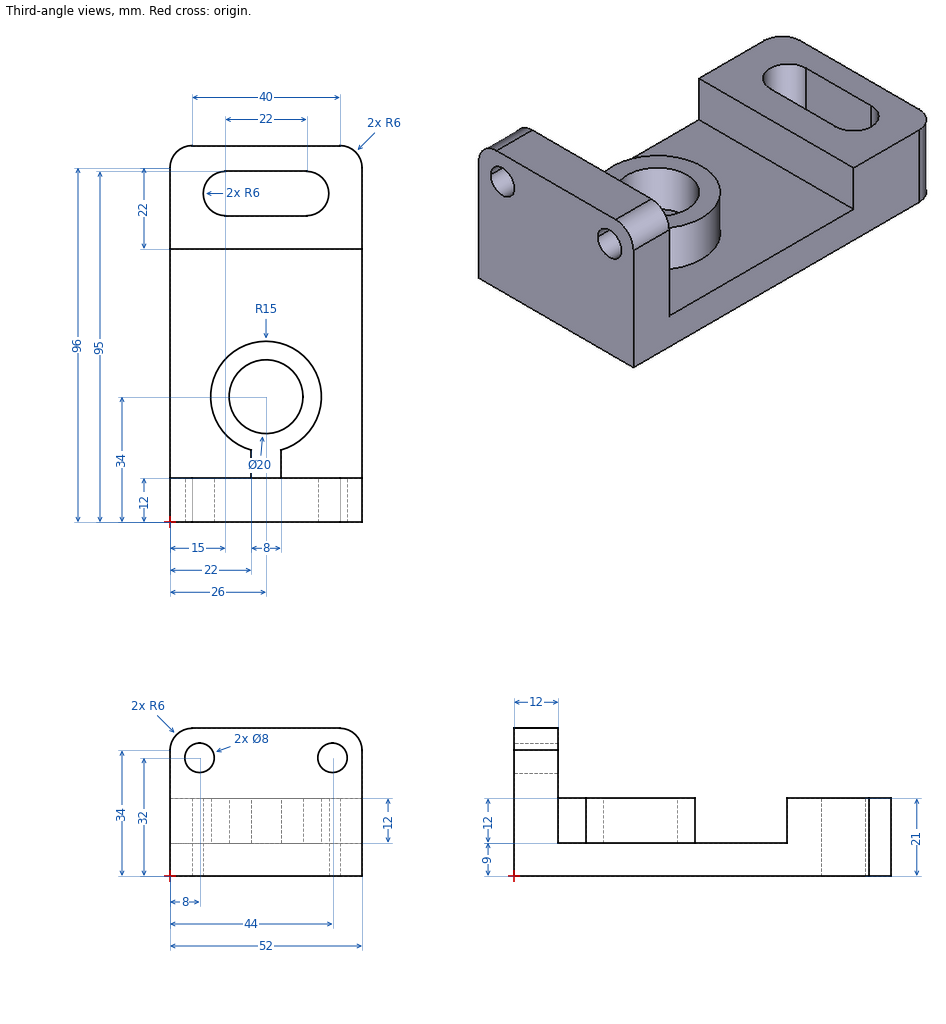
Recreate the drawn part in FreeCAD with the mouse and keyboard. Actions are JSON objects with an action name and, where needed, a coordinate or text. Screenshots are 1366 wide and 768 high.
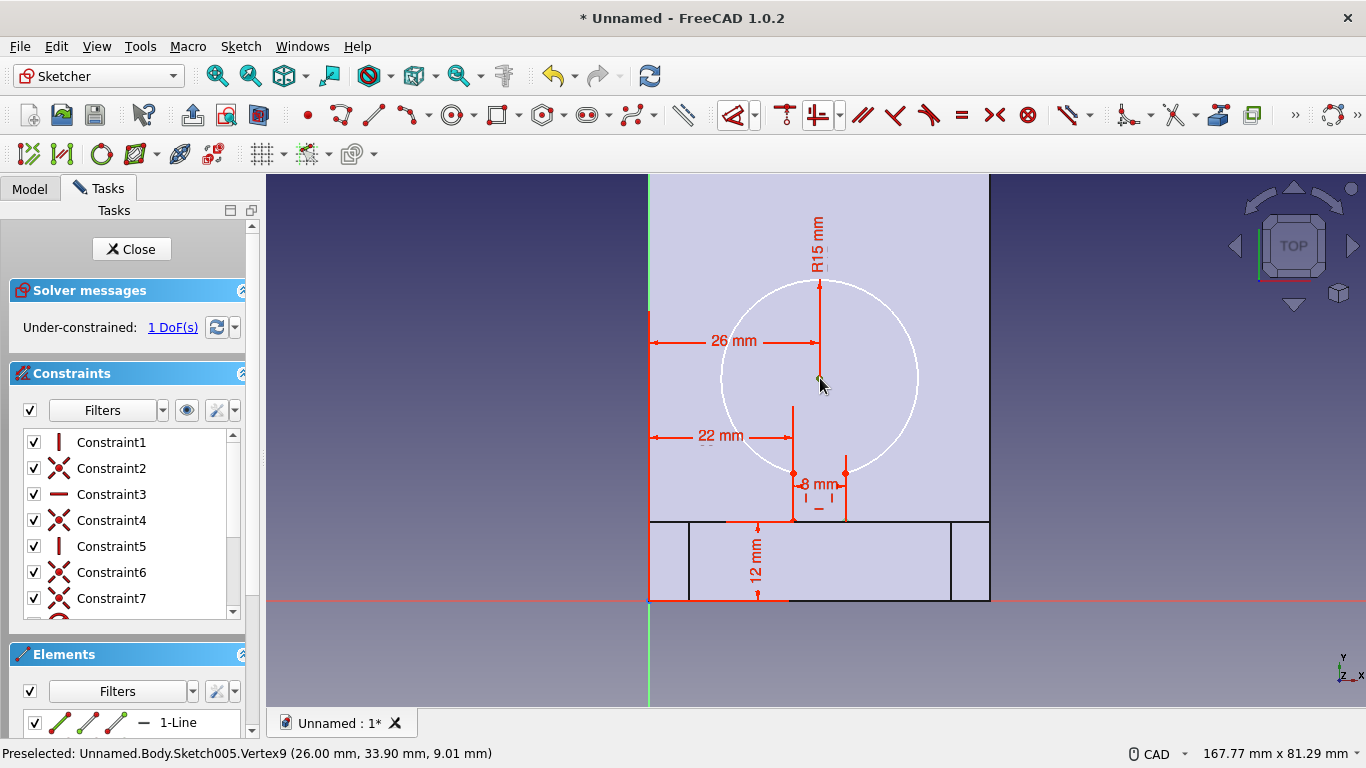
{"action": "left_click", "coordinate": [754, 116]}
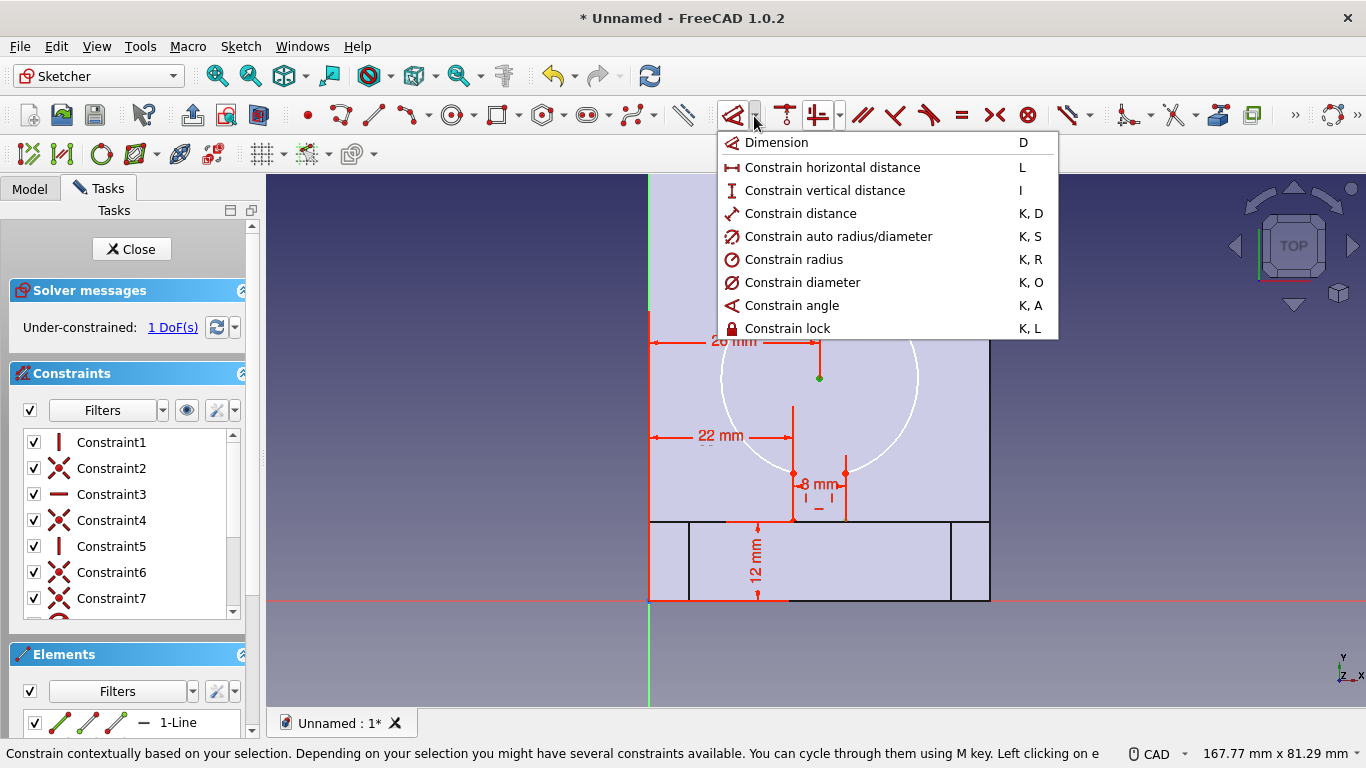
{"action": "left_click", "coordinate": [888, 190]}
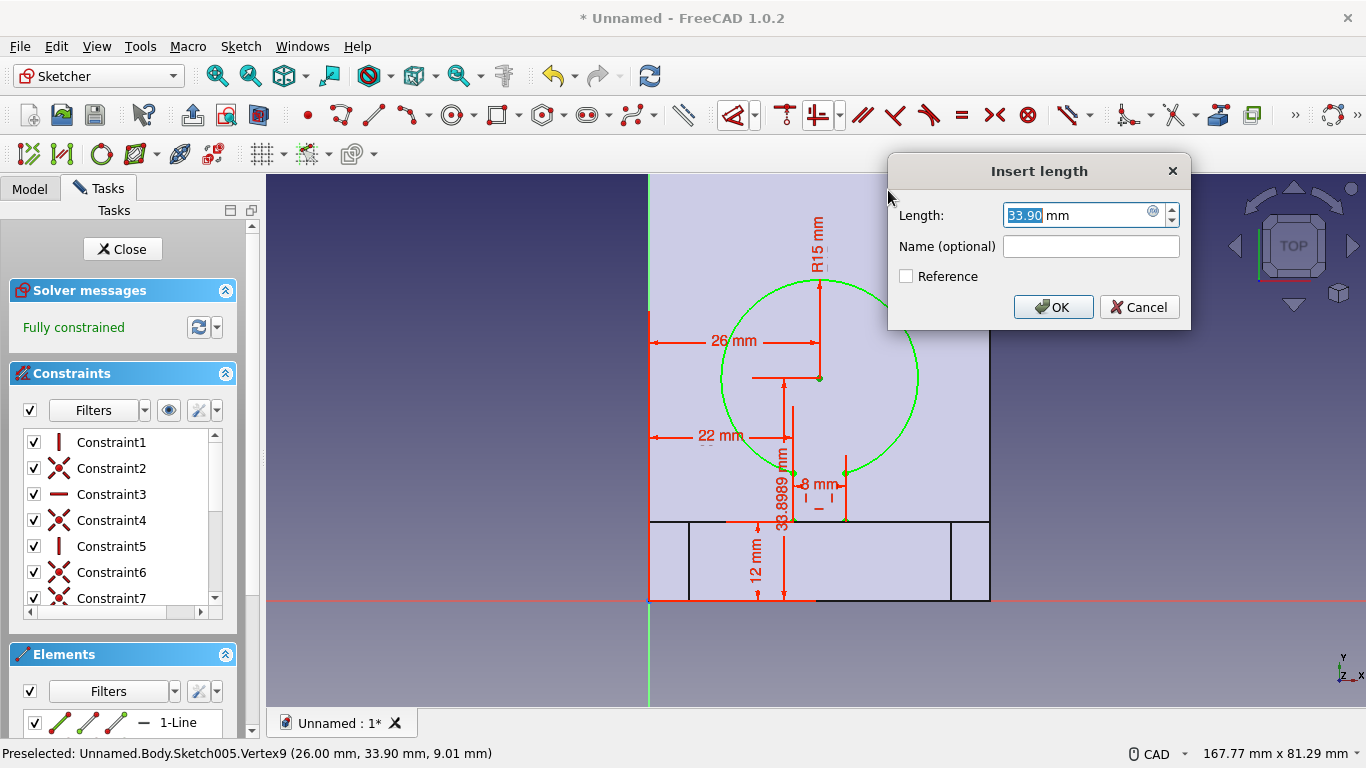
{"action": "type", "text": "34"}
{"action": "key", "text": "Return"}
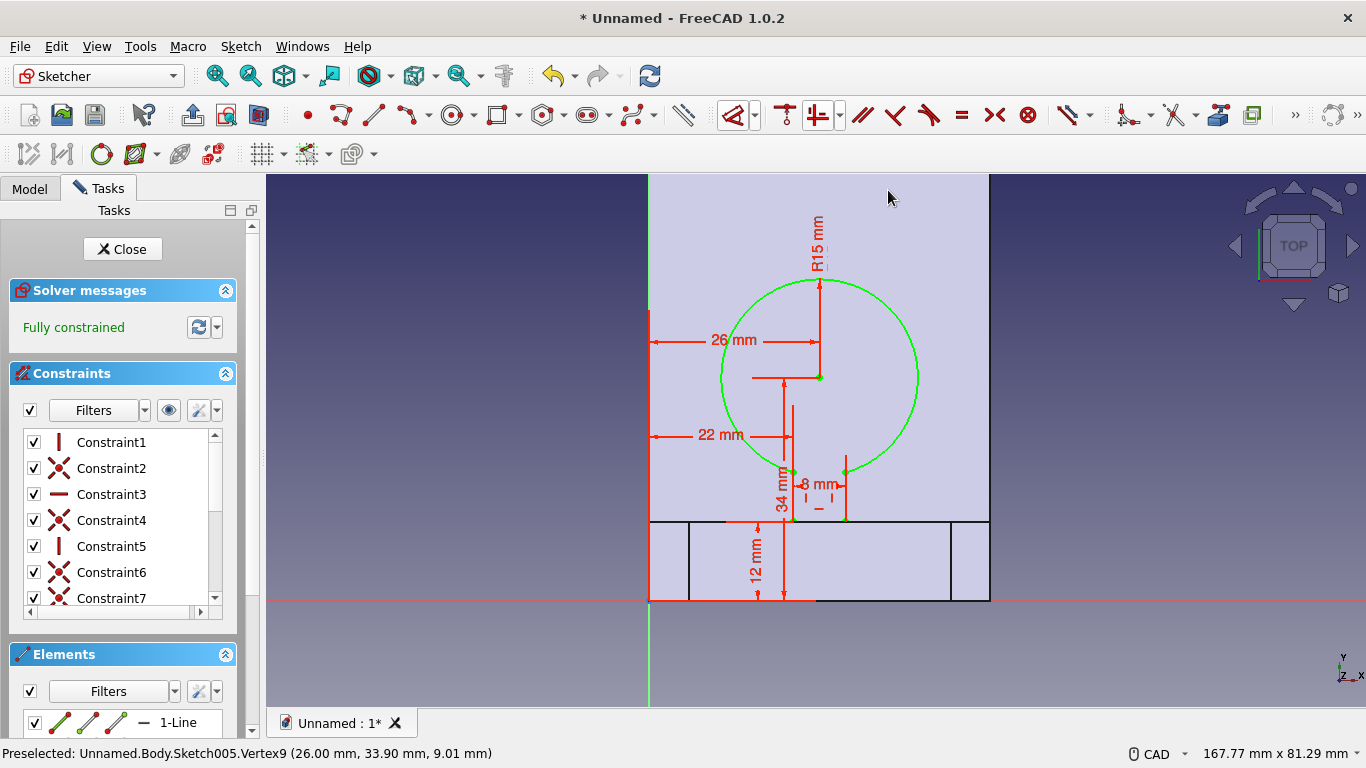
{"action": "left_click", "coordinate": [123, 249]}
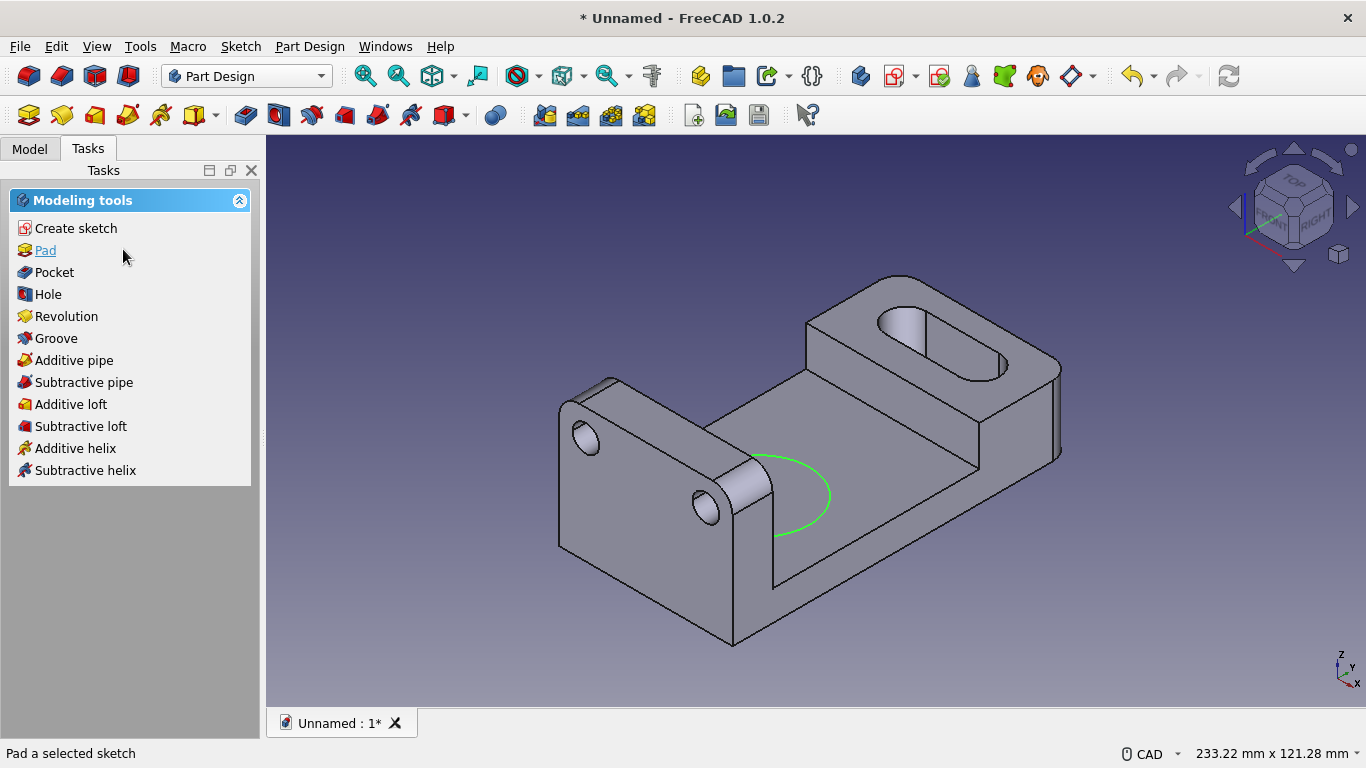
{"action": "left_click", "coordinate": [29, 116]}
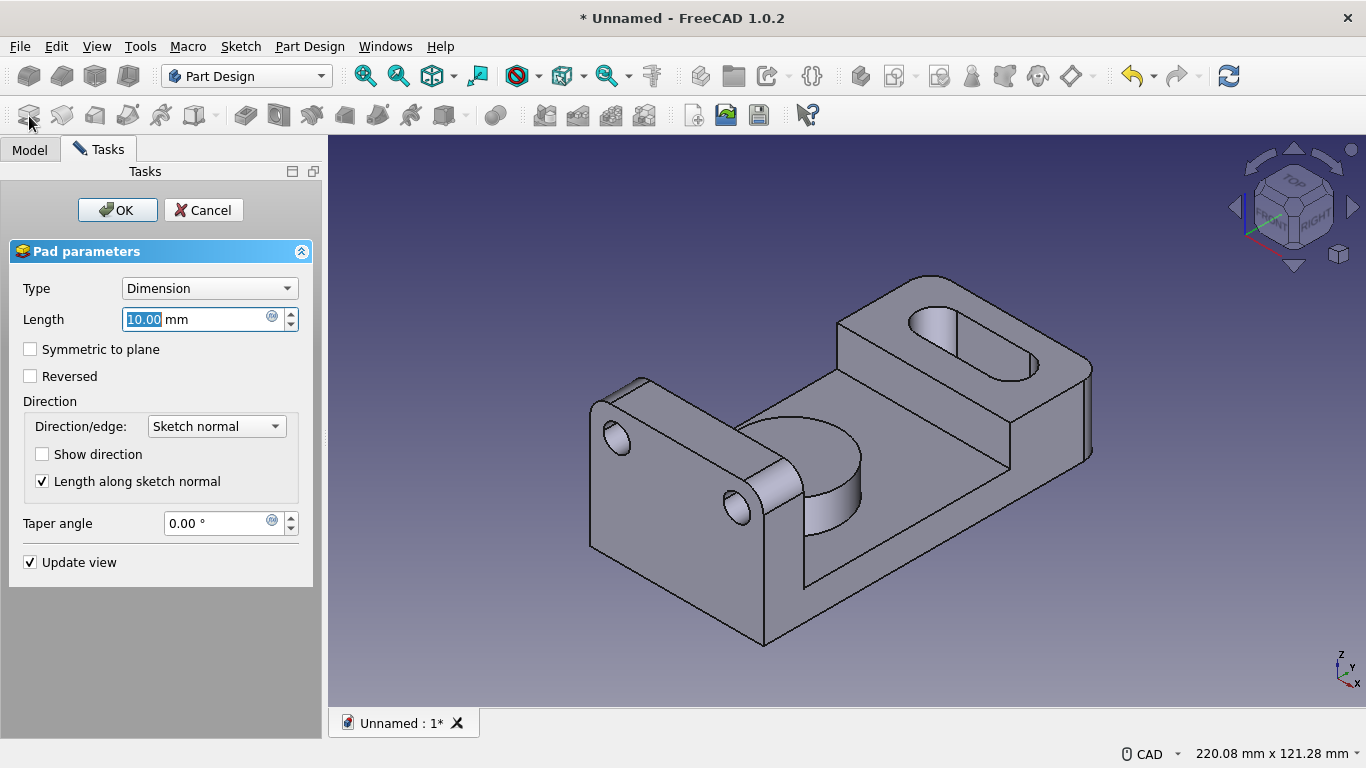
{"action": "type", "text": "12"}
{"action": "key", "text": "Tab"}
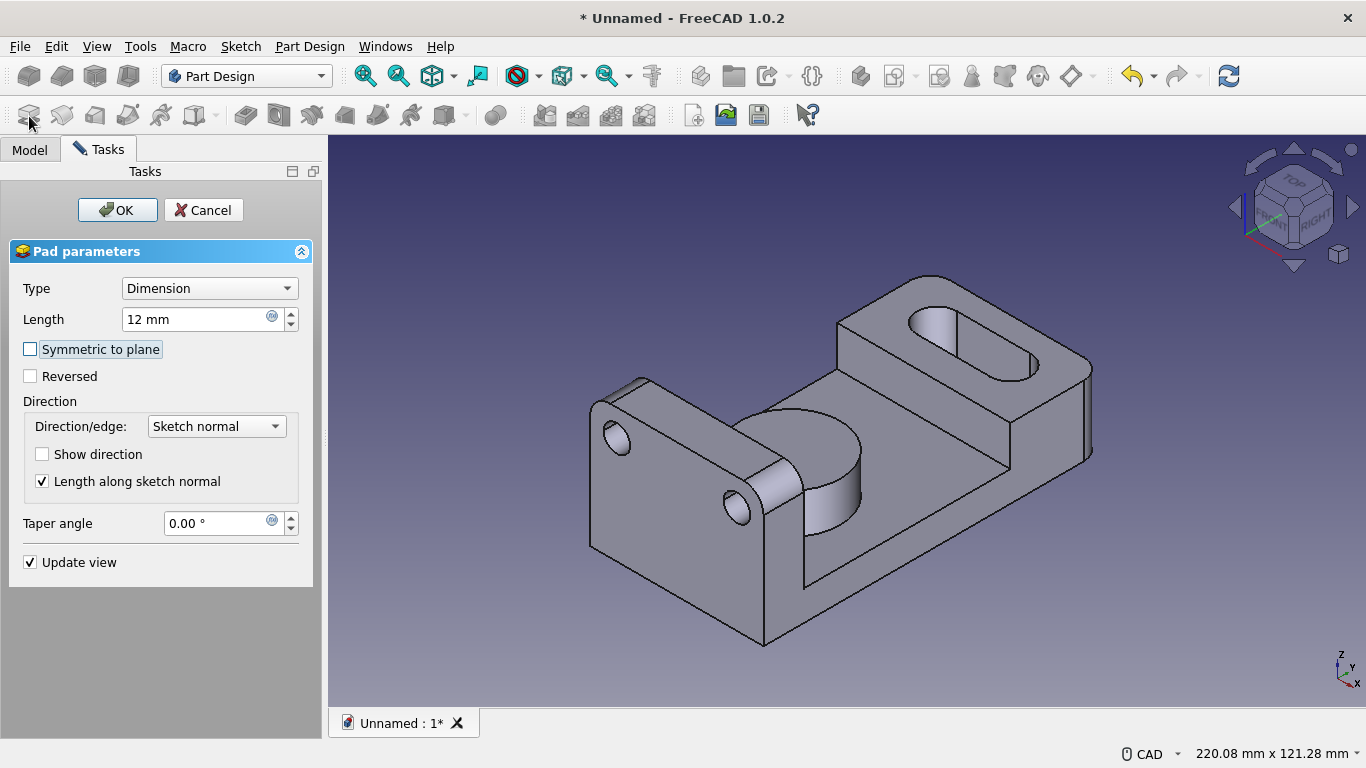
{"action": "left_click", "coordinate": [118, 210]}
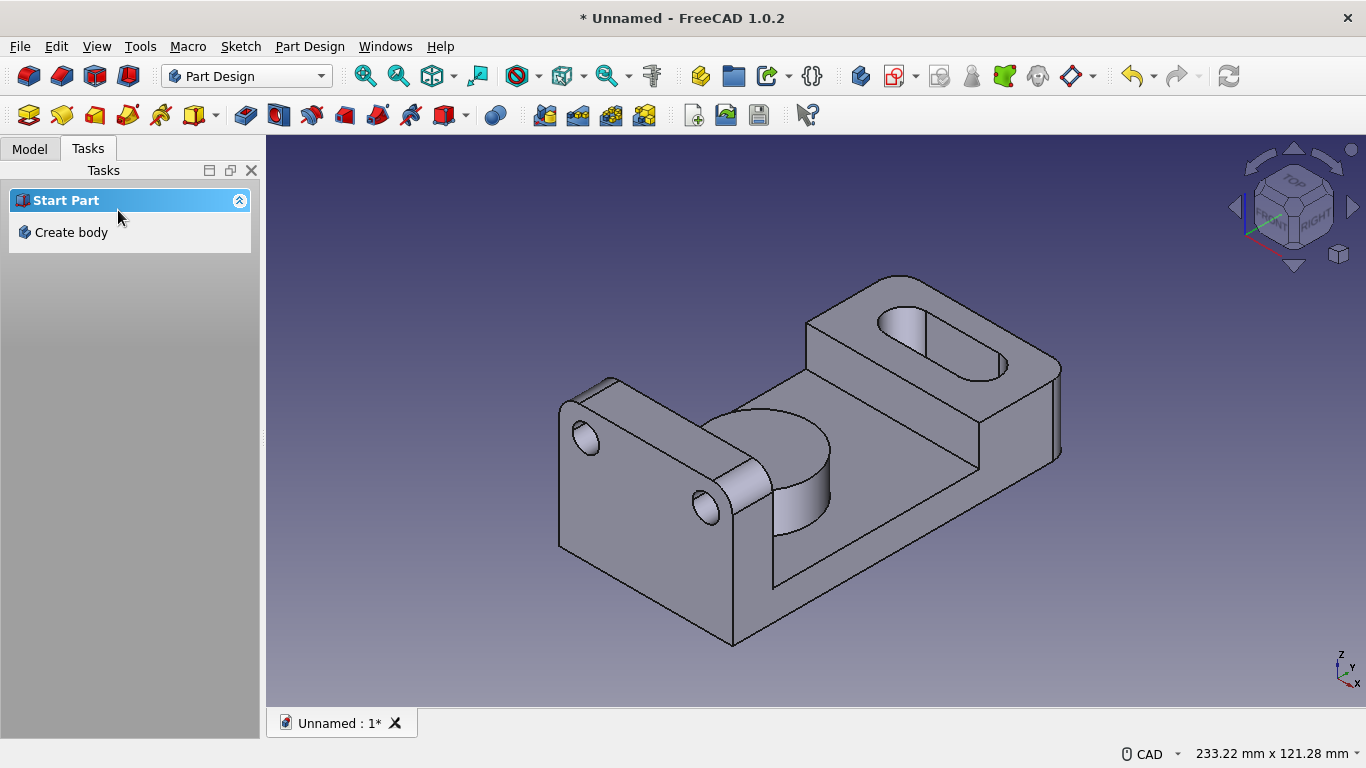
{"action": "left_click", "coordinate": [962, 389]}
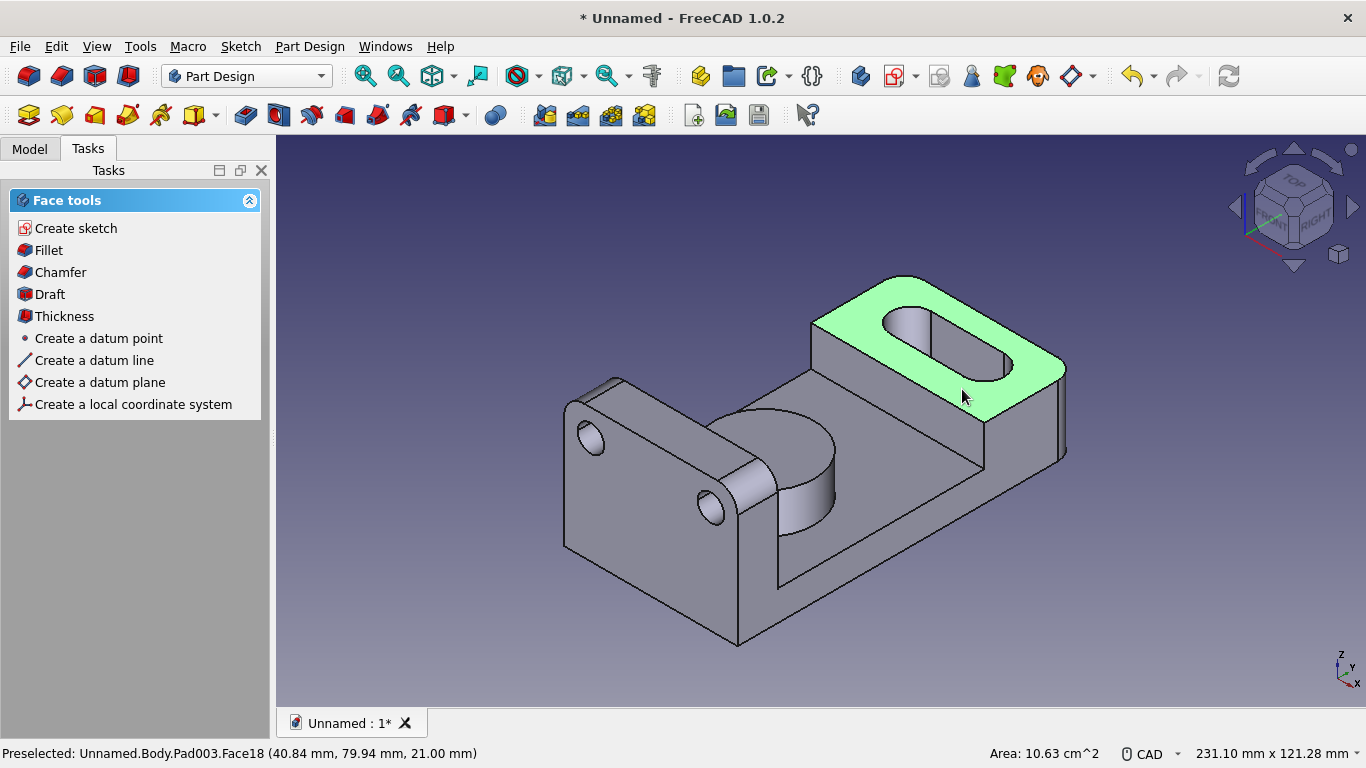
{"action": "left_click", "coordinate": [894, 76]}